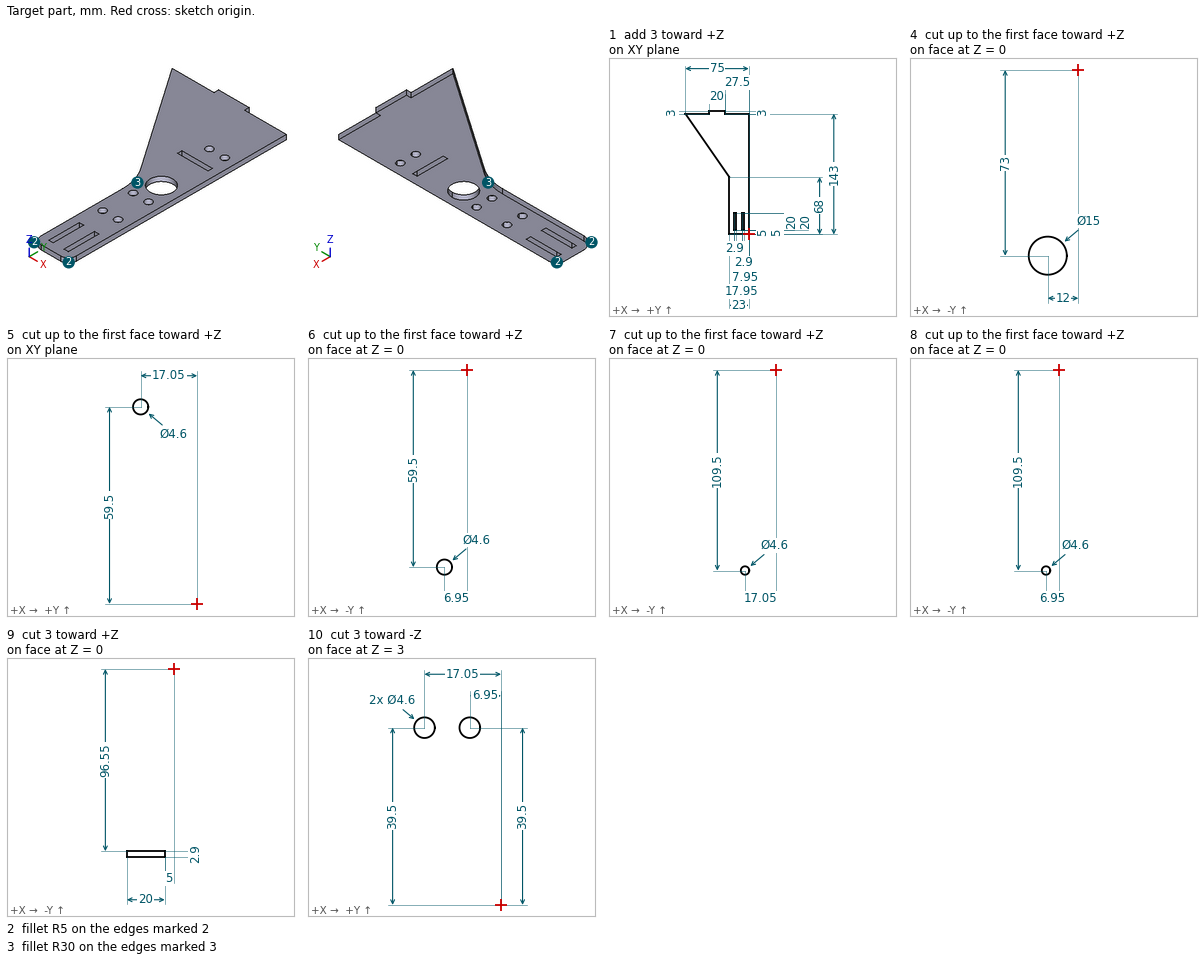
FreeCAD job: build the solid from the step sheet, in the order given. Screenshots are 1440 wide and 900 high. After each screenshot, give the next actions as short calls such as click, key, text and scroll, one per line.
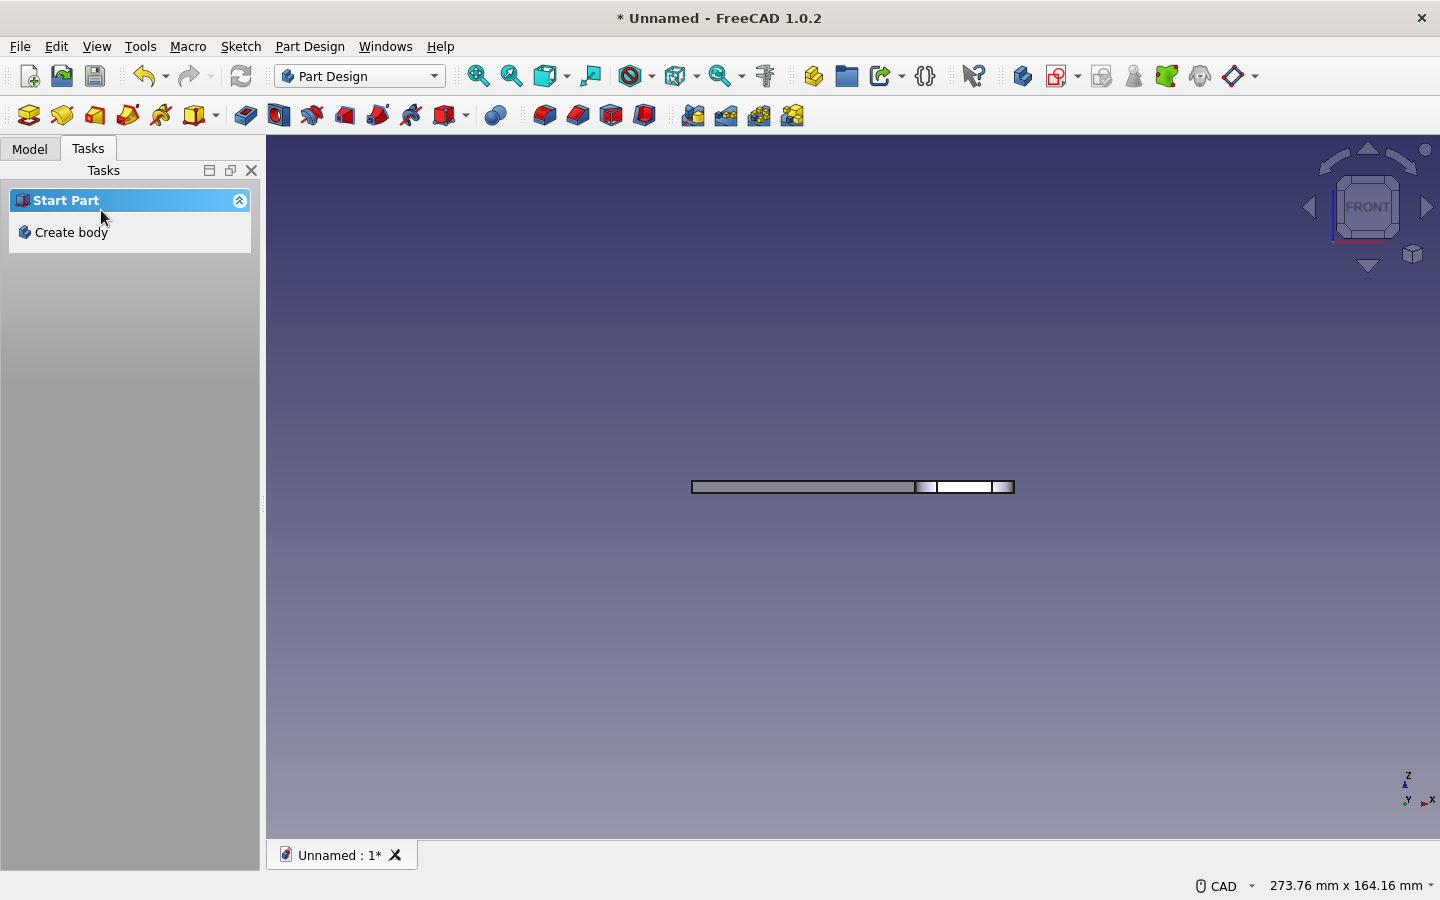
key(v)
key(f)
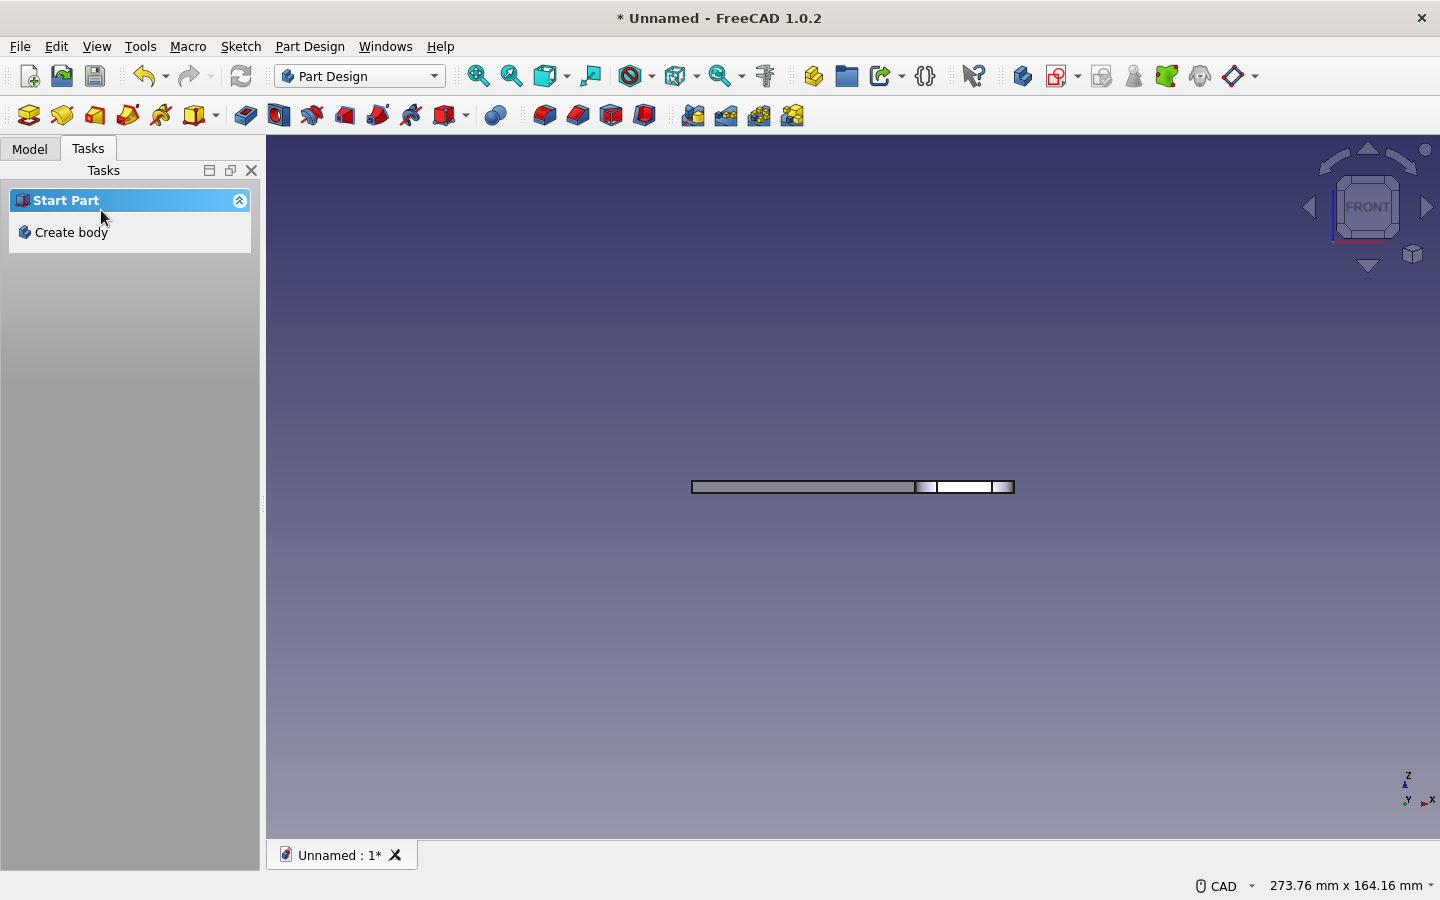
scroll(915, 486, up, 6)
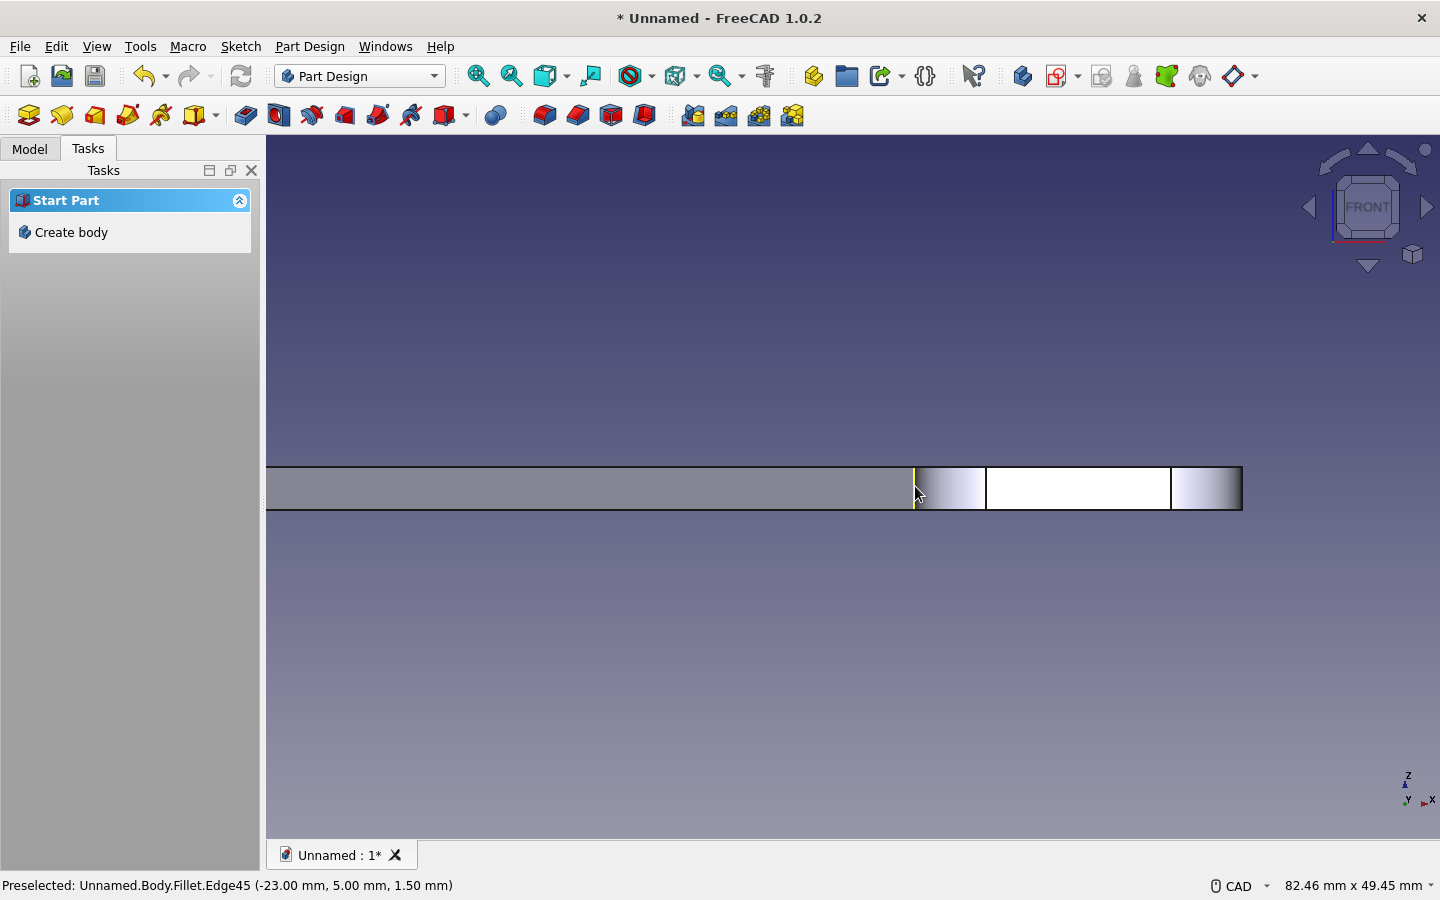
click(479, 76)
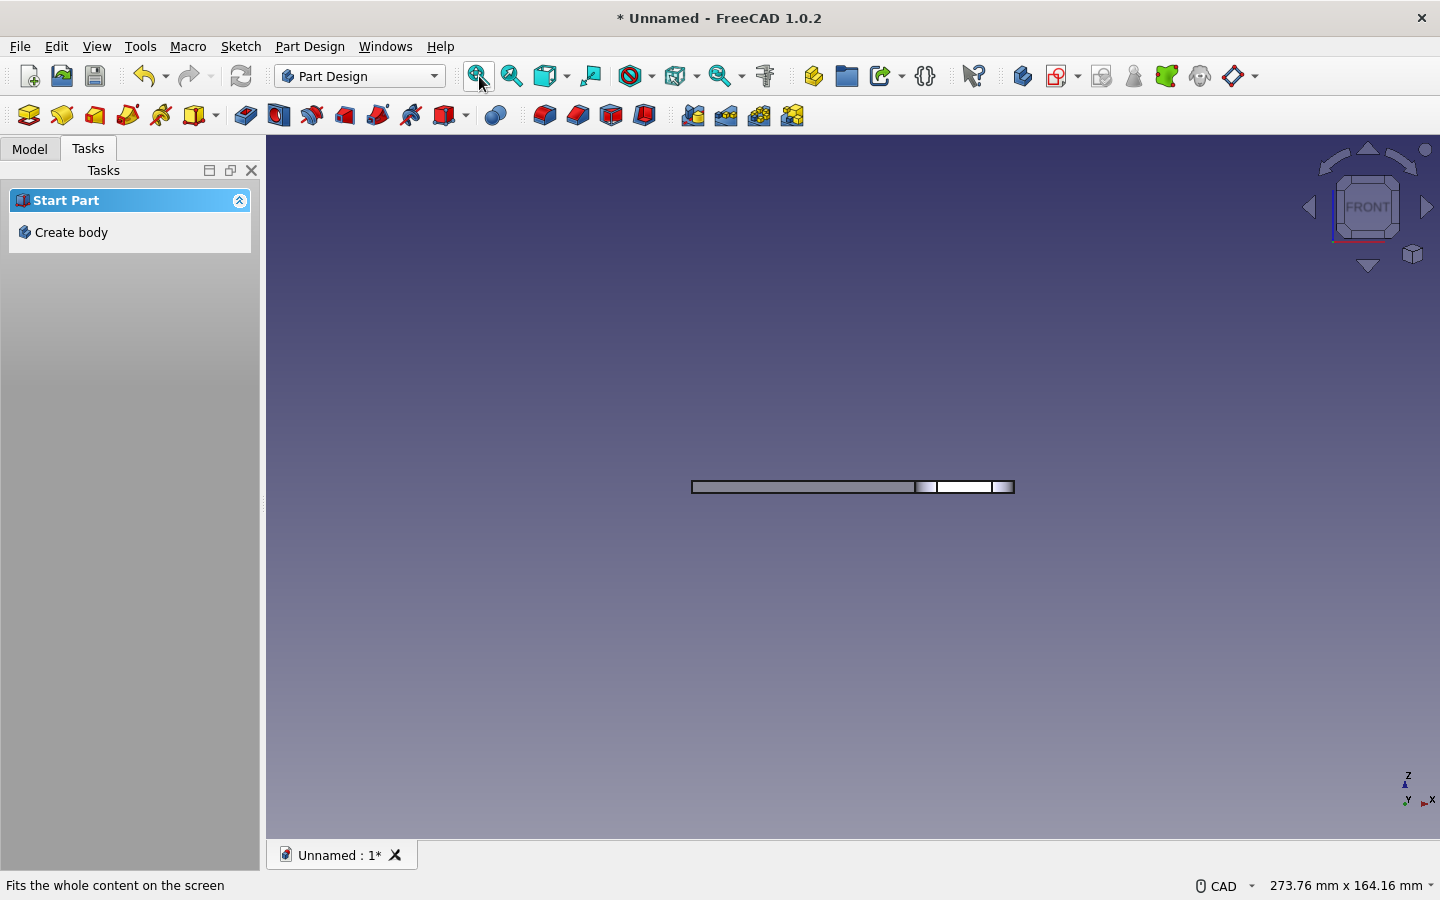
key(0)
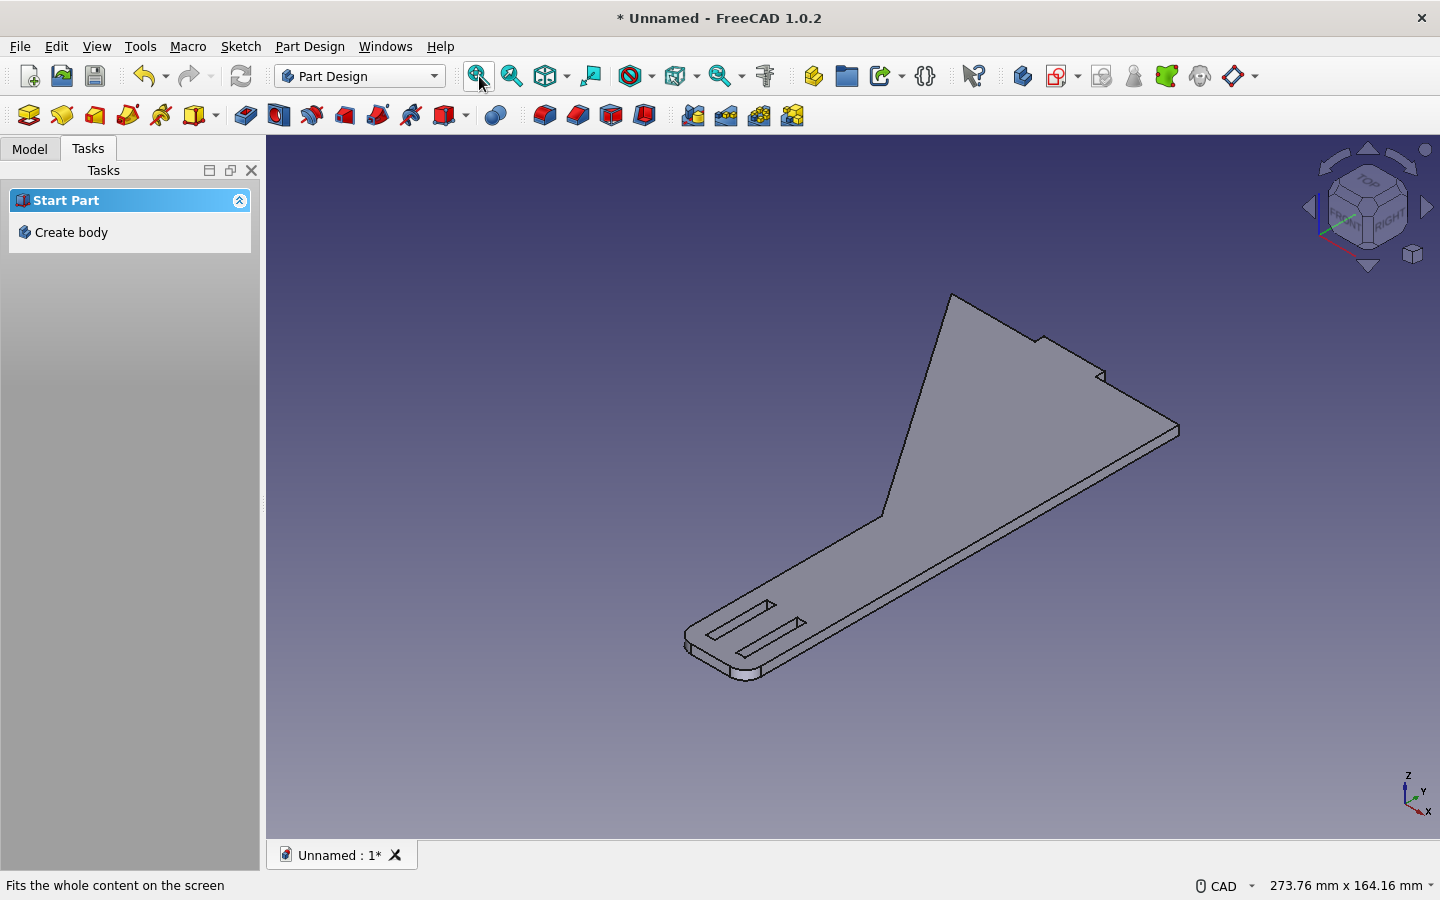
scroll(882, 520, up, 6)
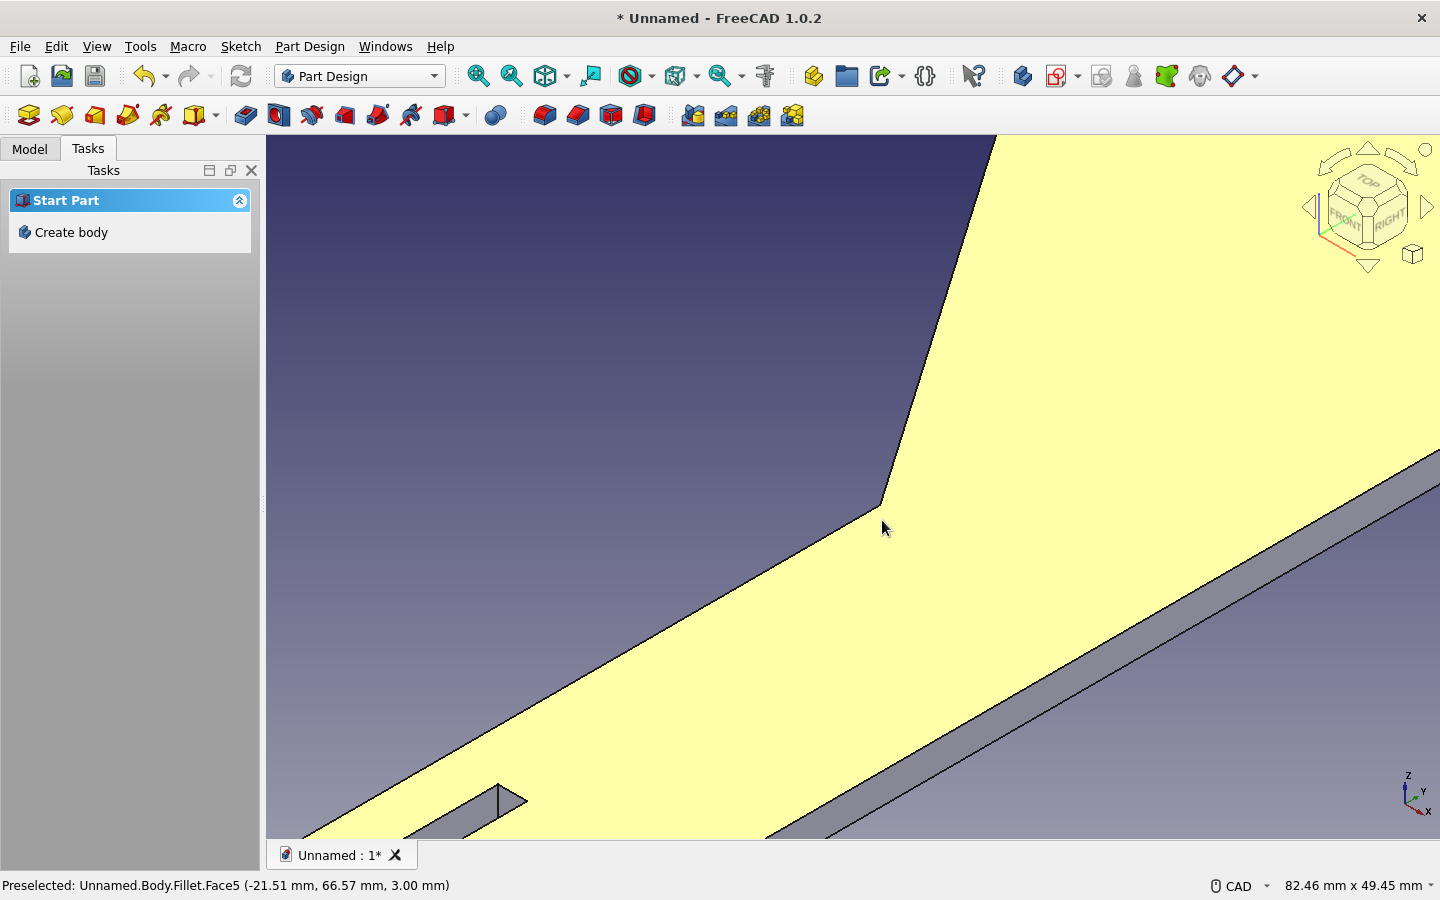
key(v)
key(f)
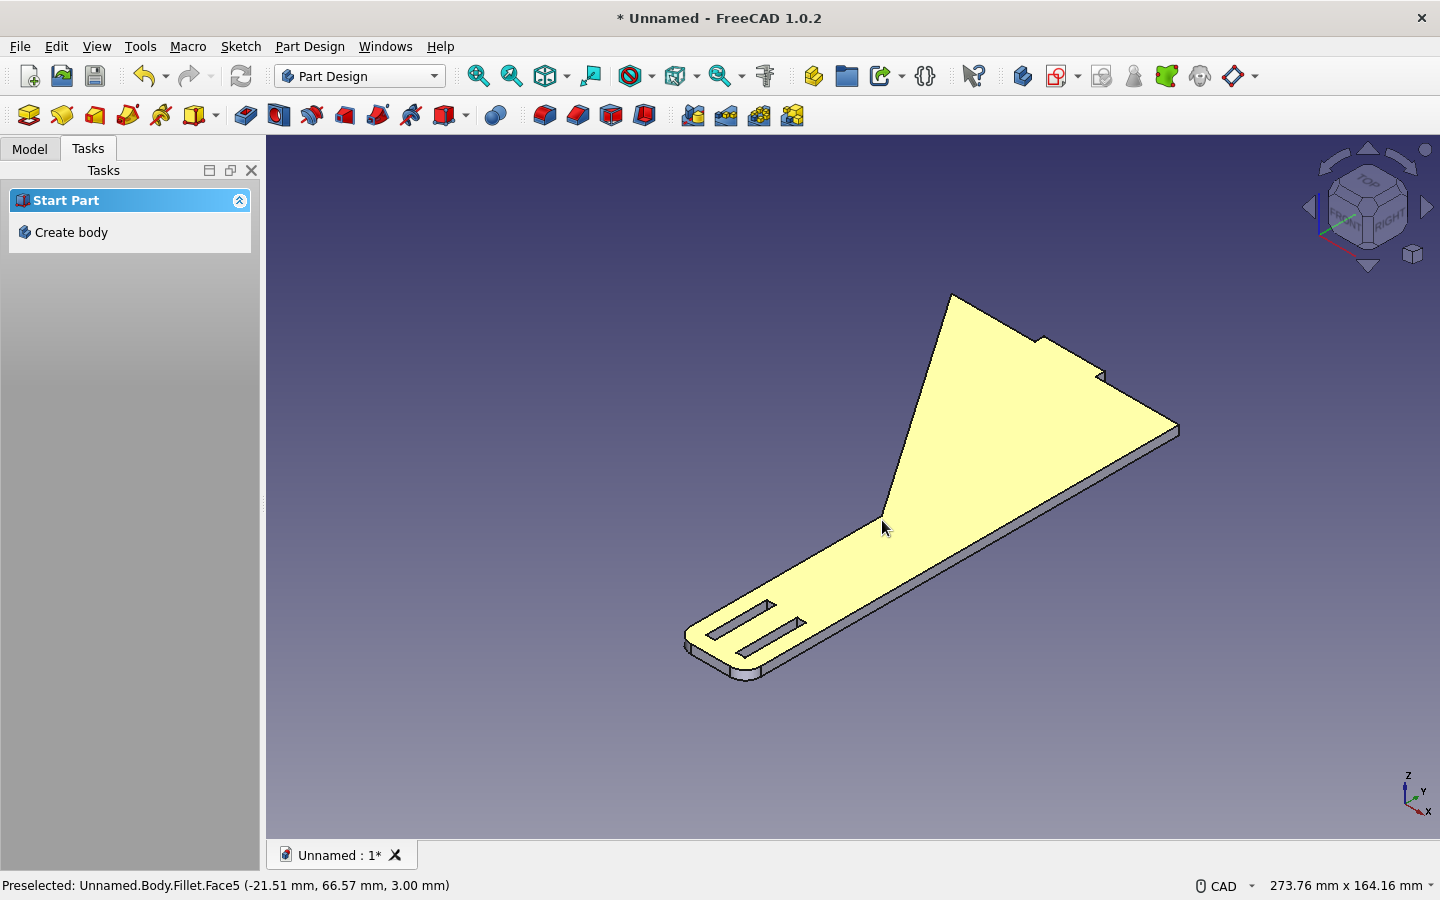
key(2)